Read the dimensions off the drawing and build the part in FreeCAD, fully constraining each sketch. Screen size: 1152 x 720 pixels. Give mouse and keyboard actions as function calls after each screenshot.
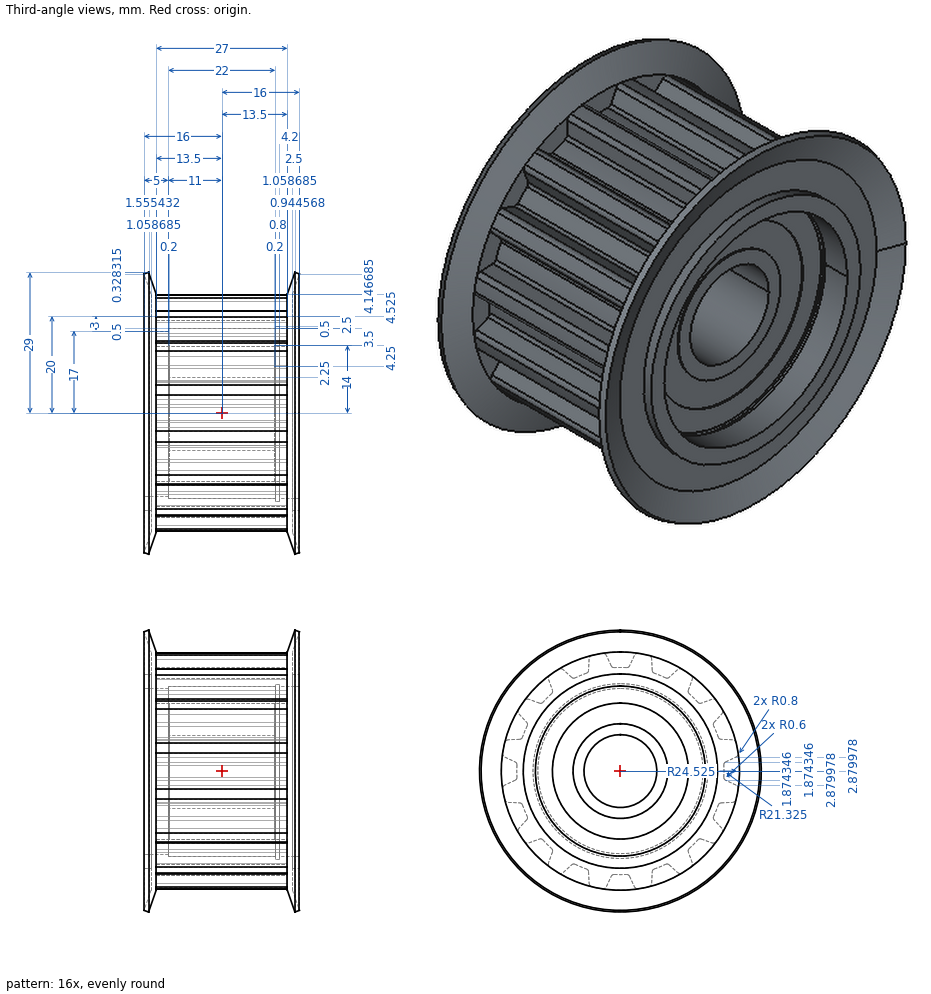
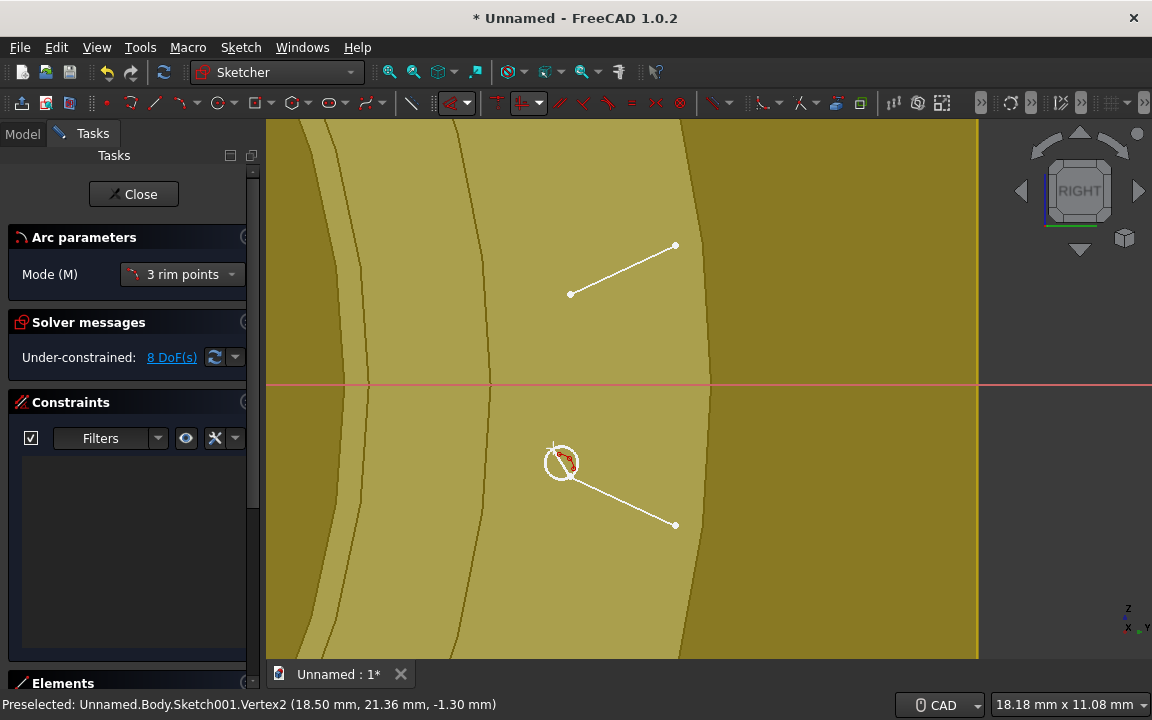
scroll(557, 465, up, 6)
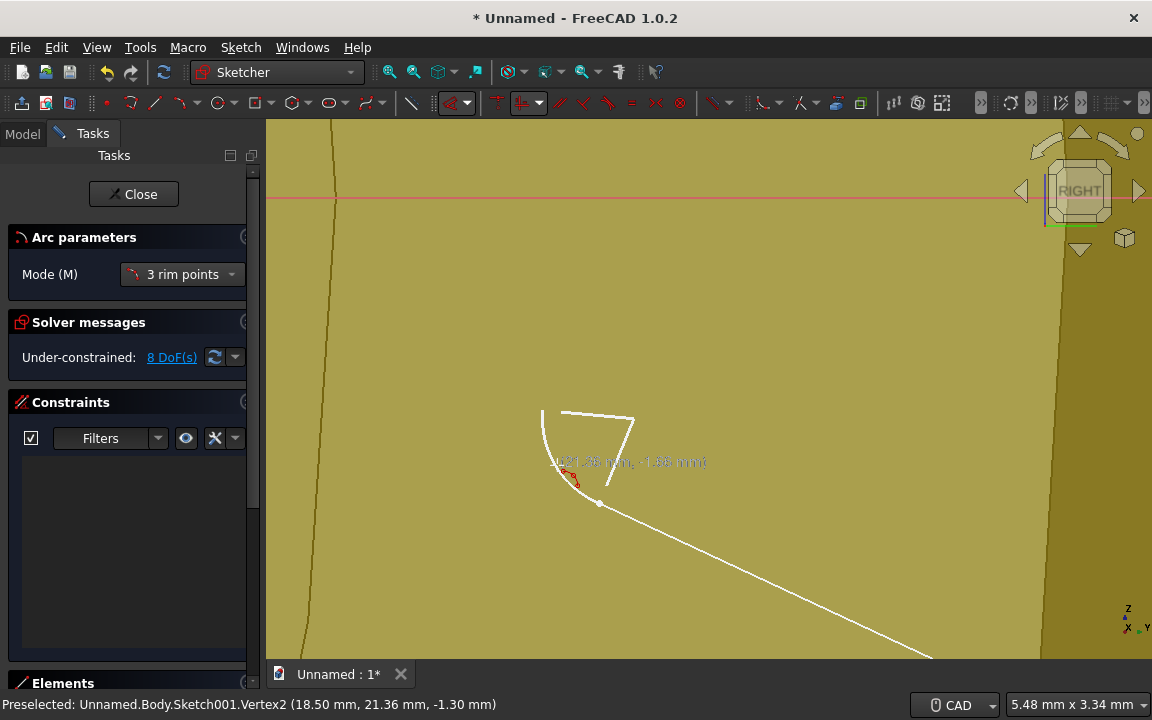
click(557, 463)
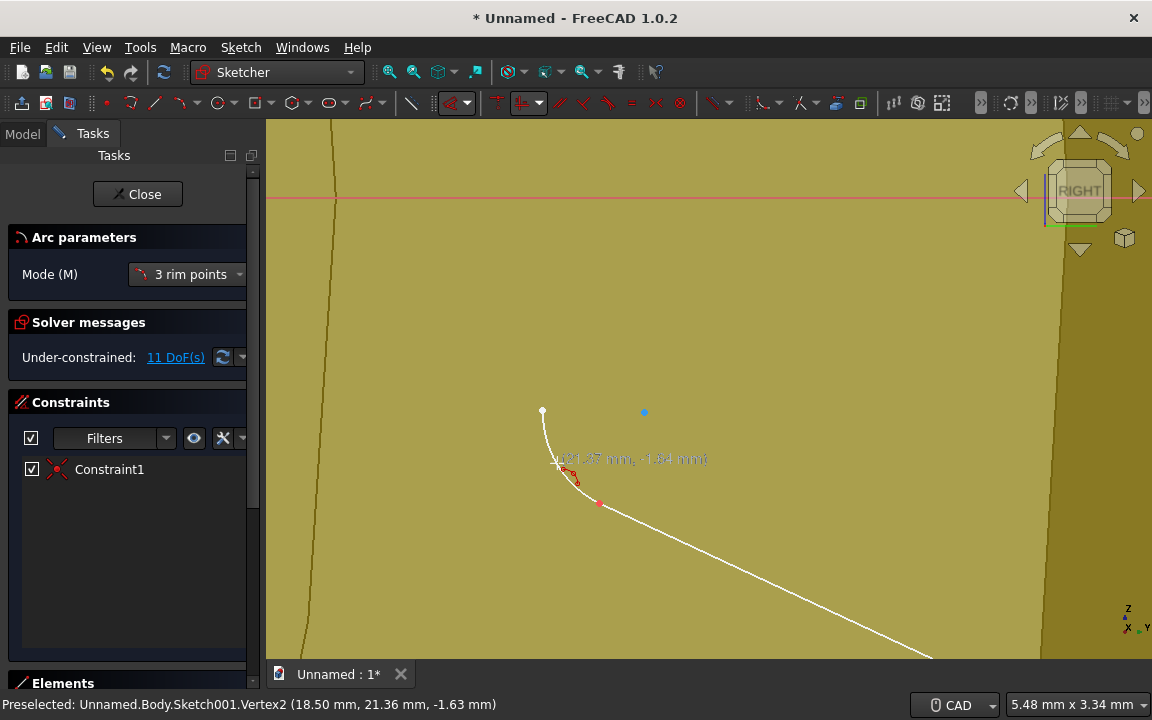
click(543, 410)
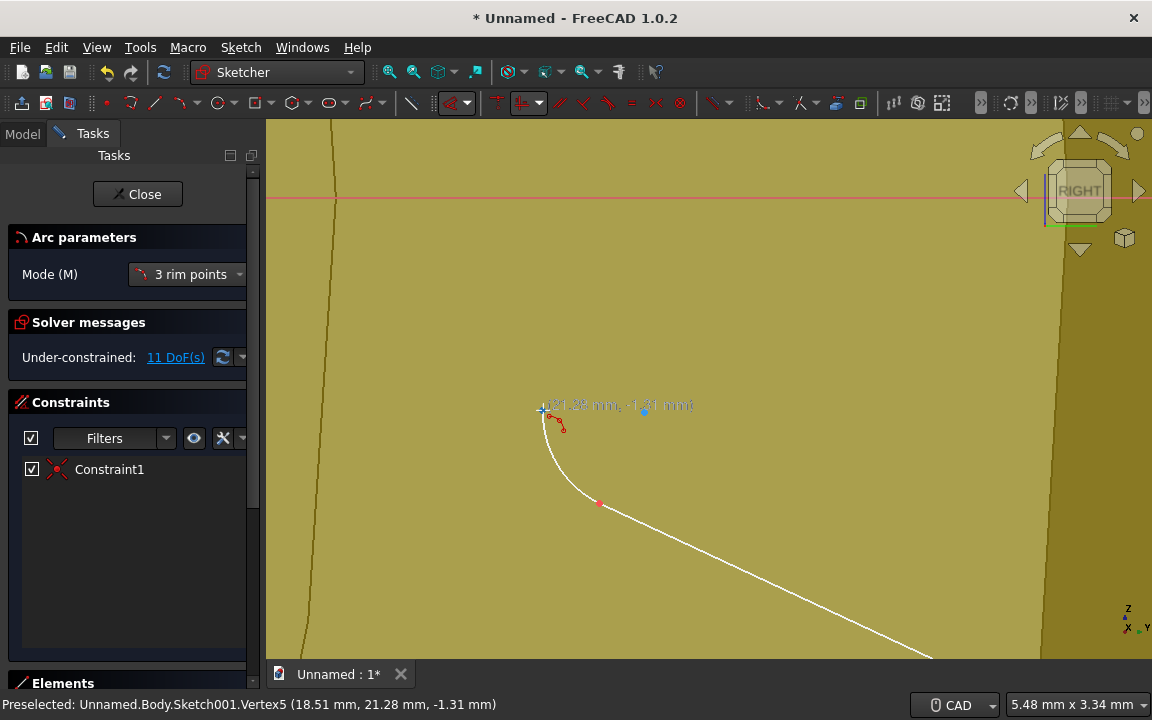
scroll(569, 471, down, 6)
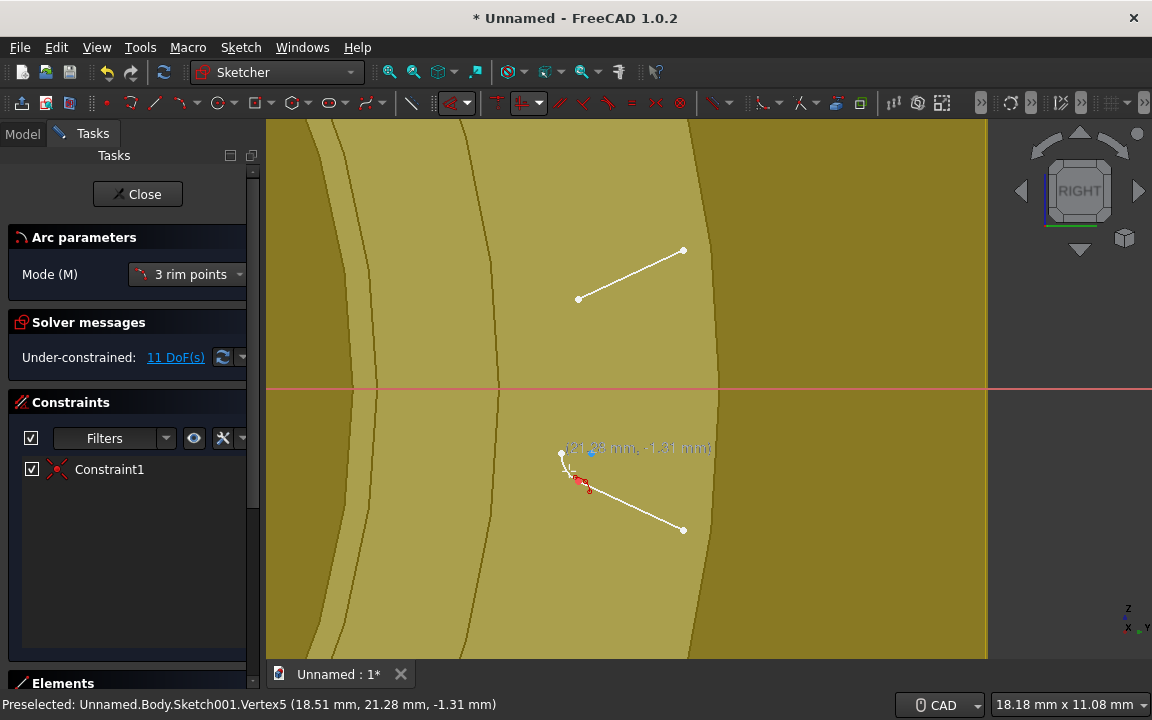
click(562, 326)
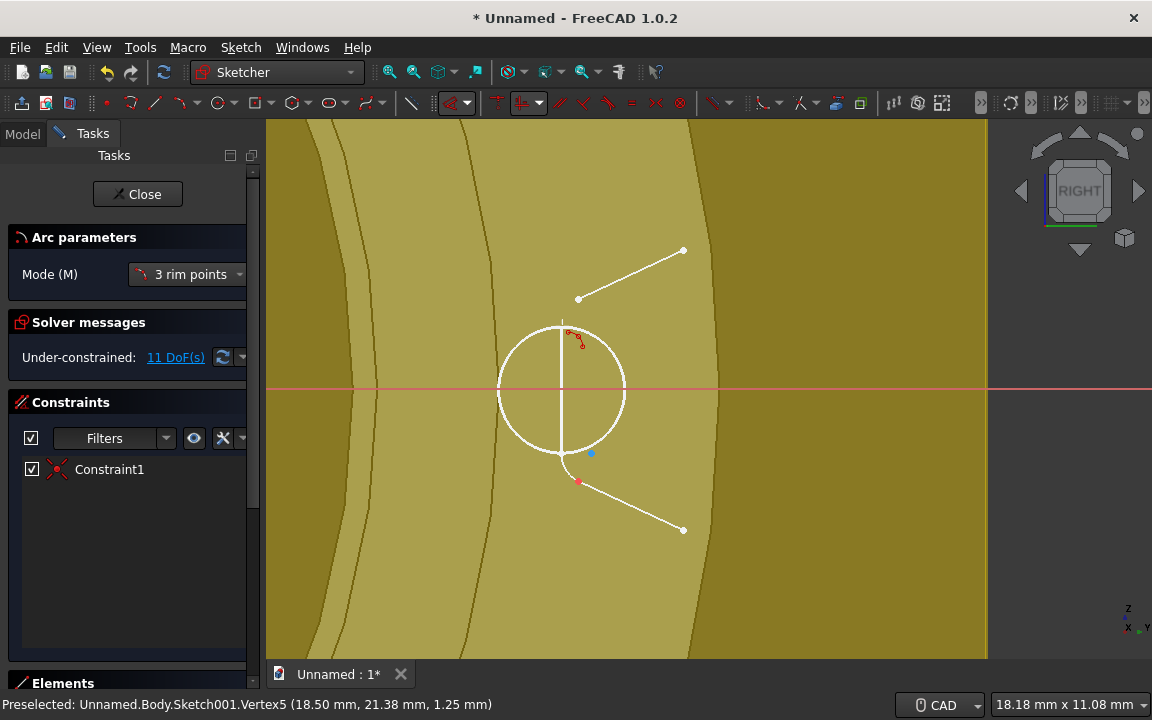
scroll(564, 402, up, 11)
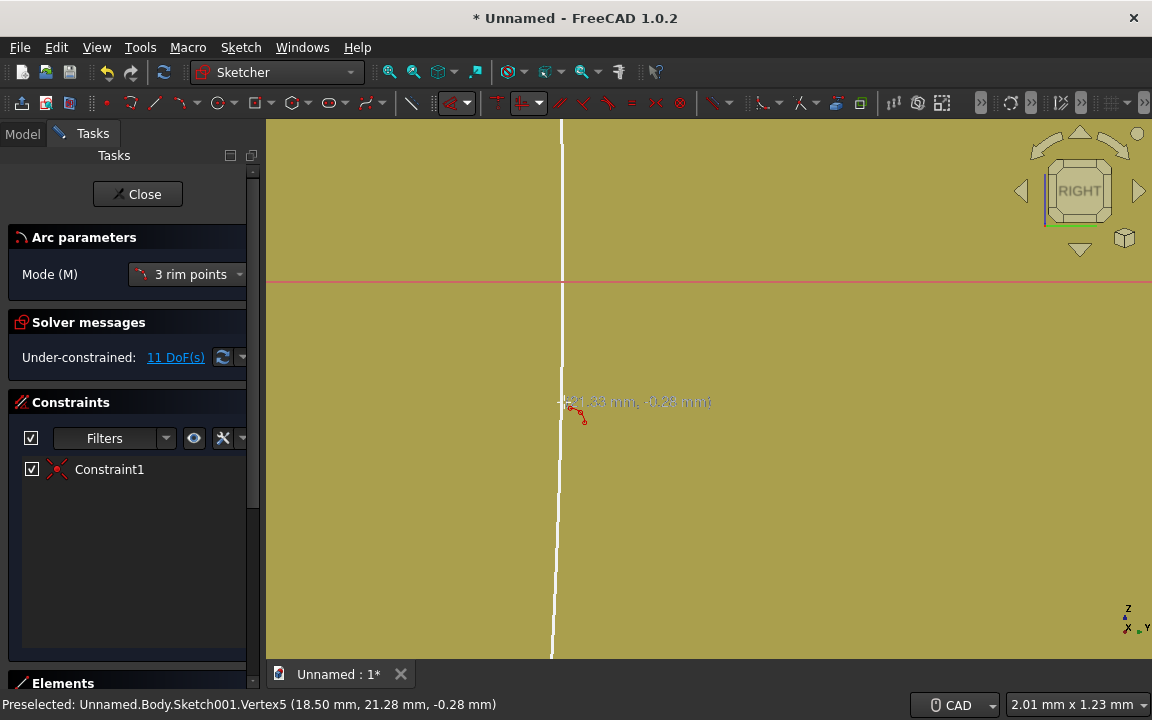
click(557, 396)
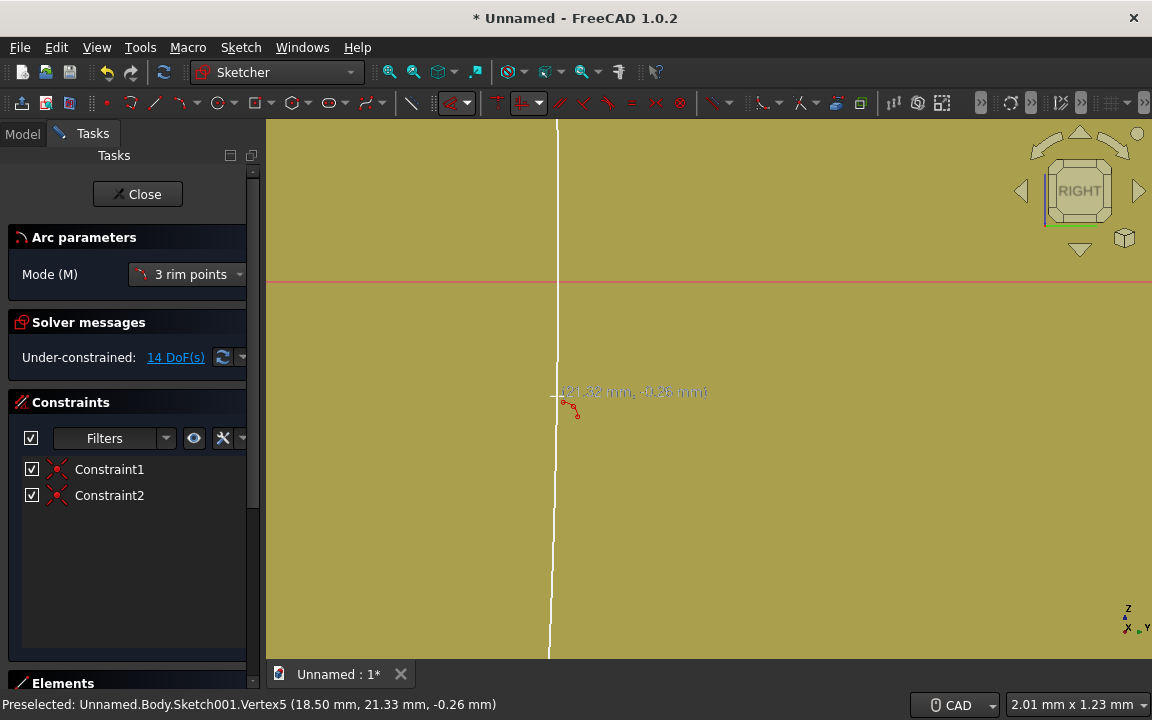
scroll(564, 402, down, 11)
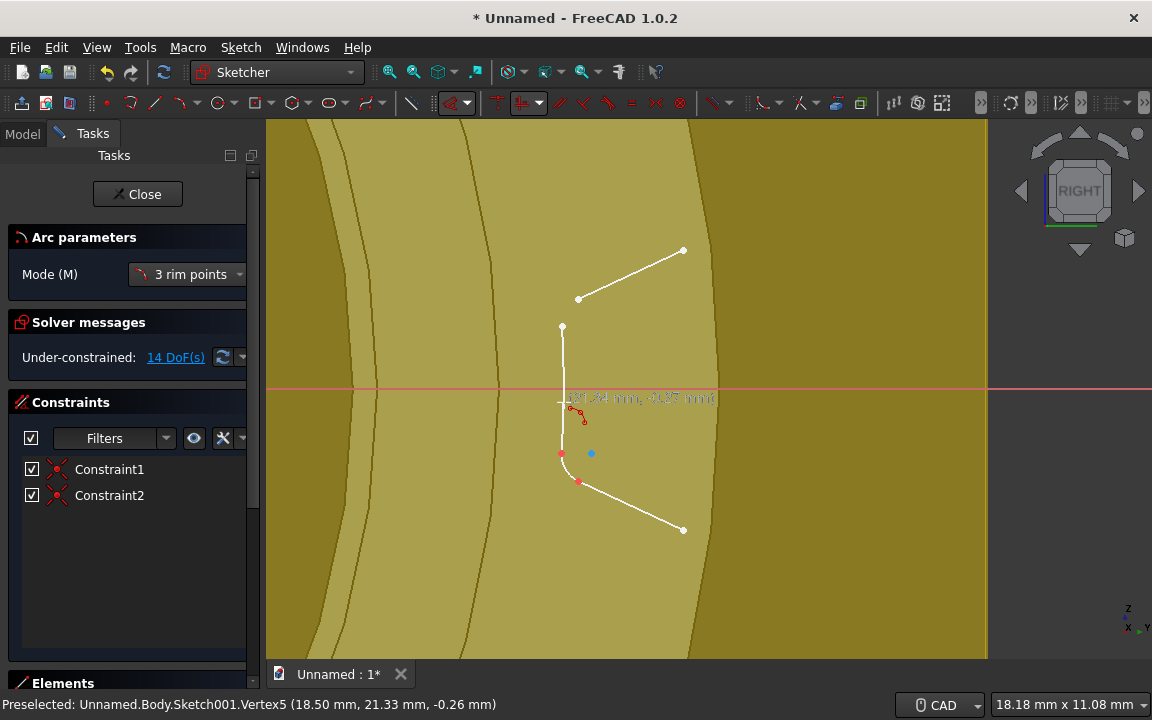
click(562, 327)
click(578, 299)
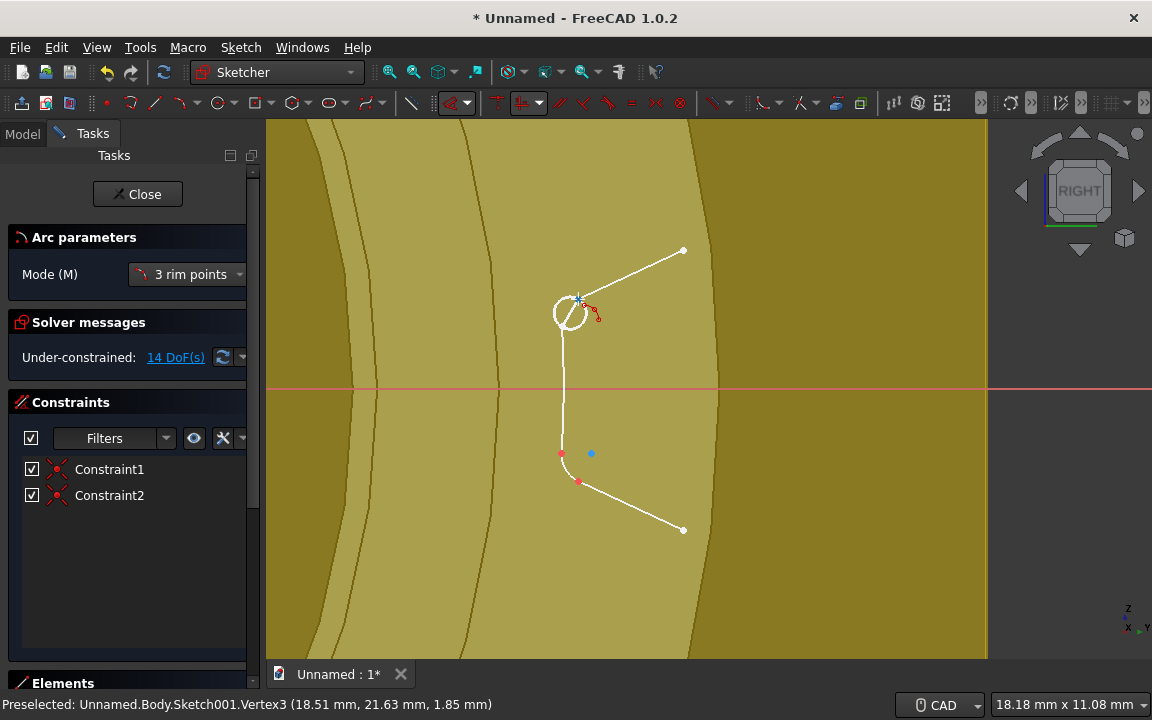
scroll(566, 309, up, 6)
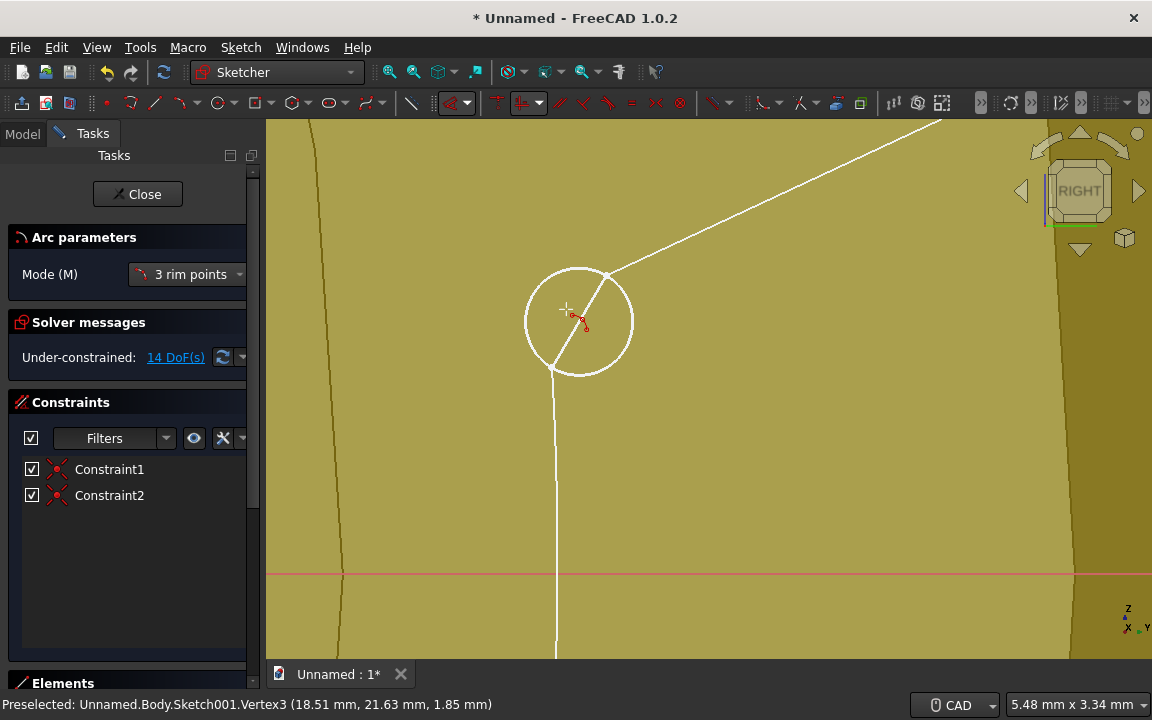
click(564, 309)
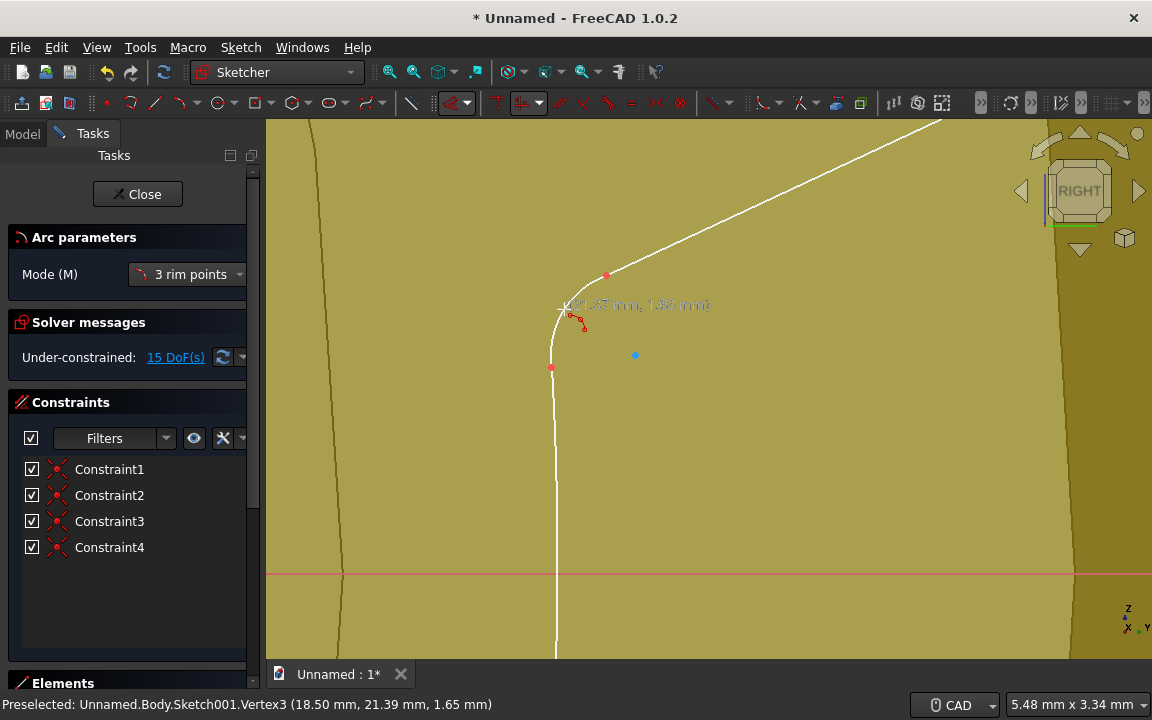
scroll(566, 309, down, 6)